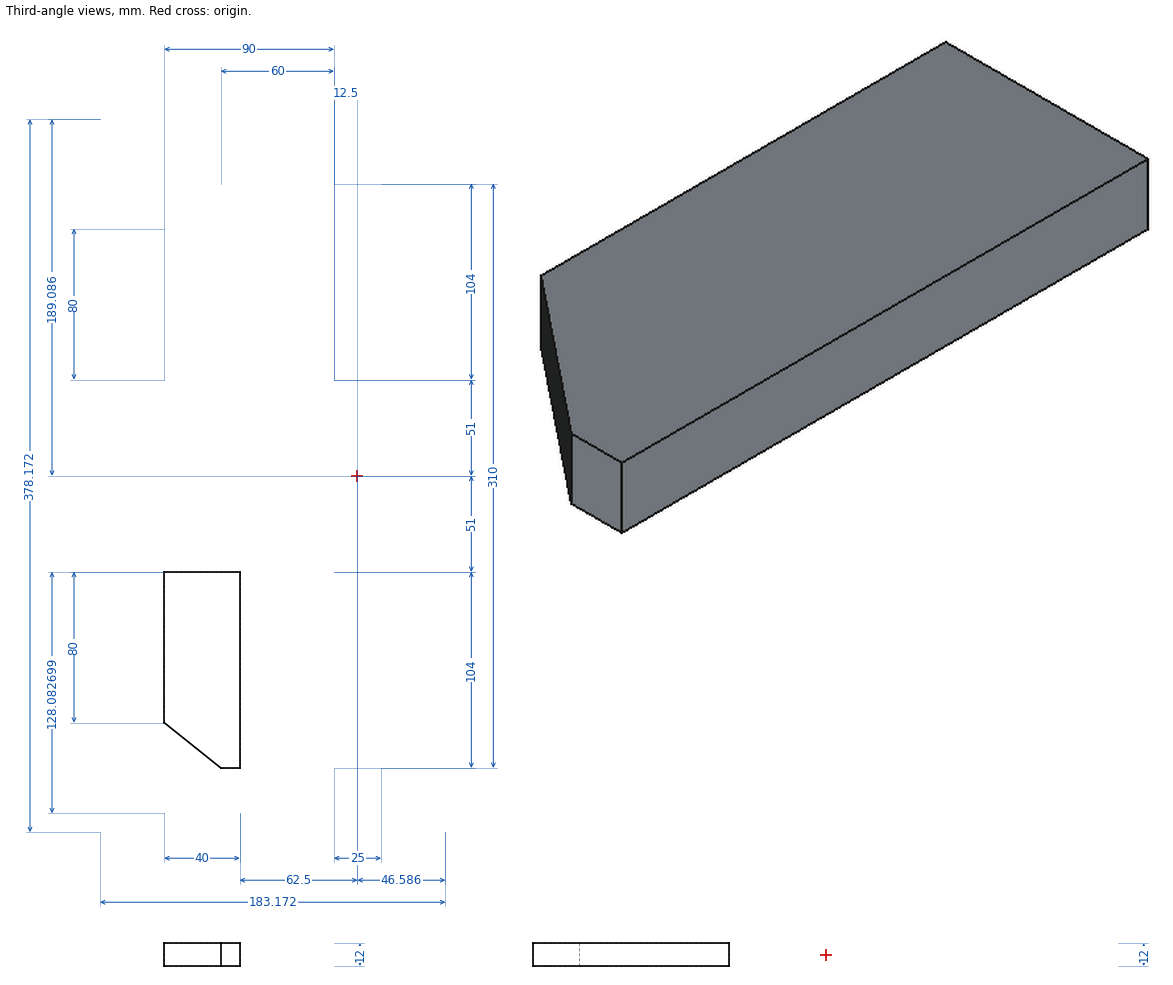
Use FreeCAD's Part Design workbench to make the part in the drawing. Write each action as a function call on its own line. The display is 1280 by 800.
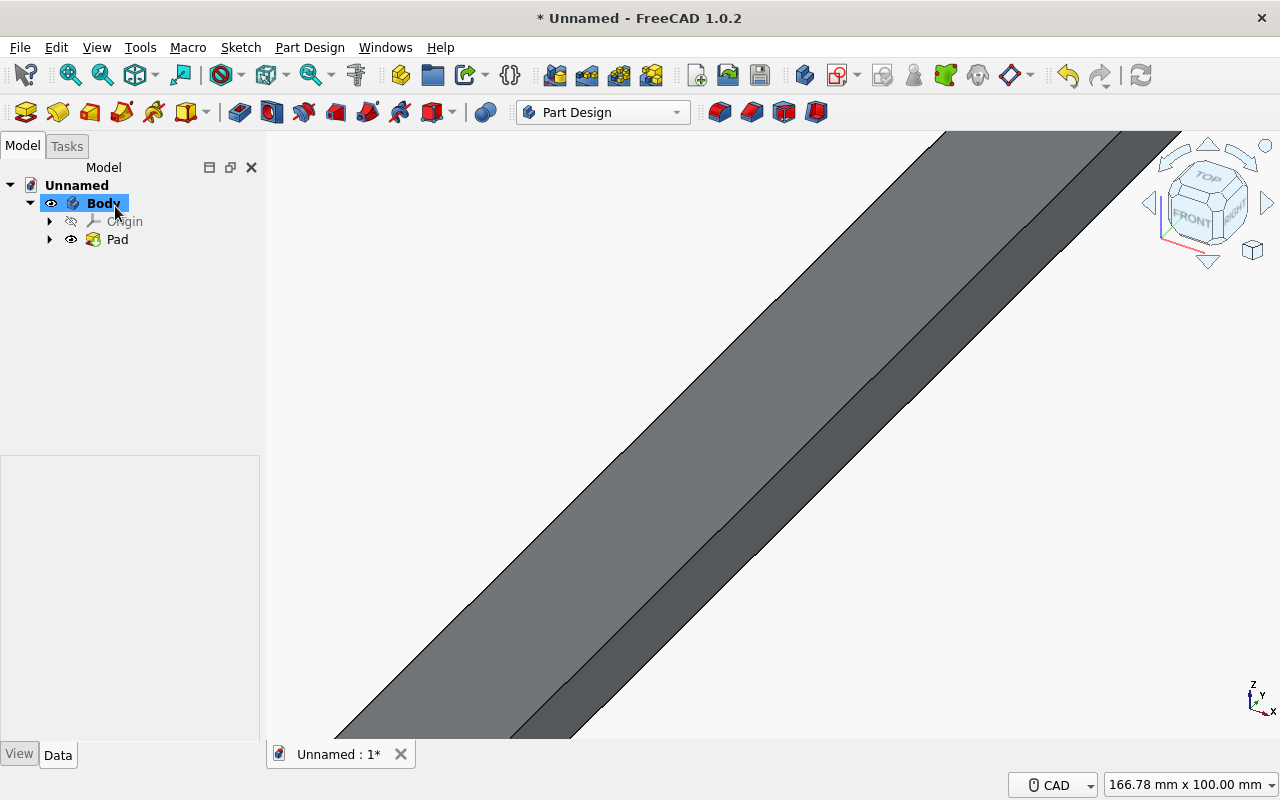
click(72, 76)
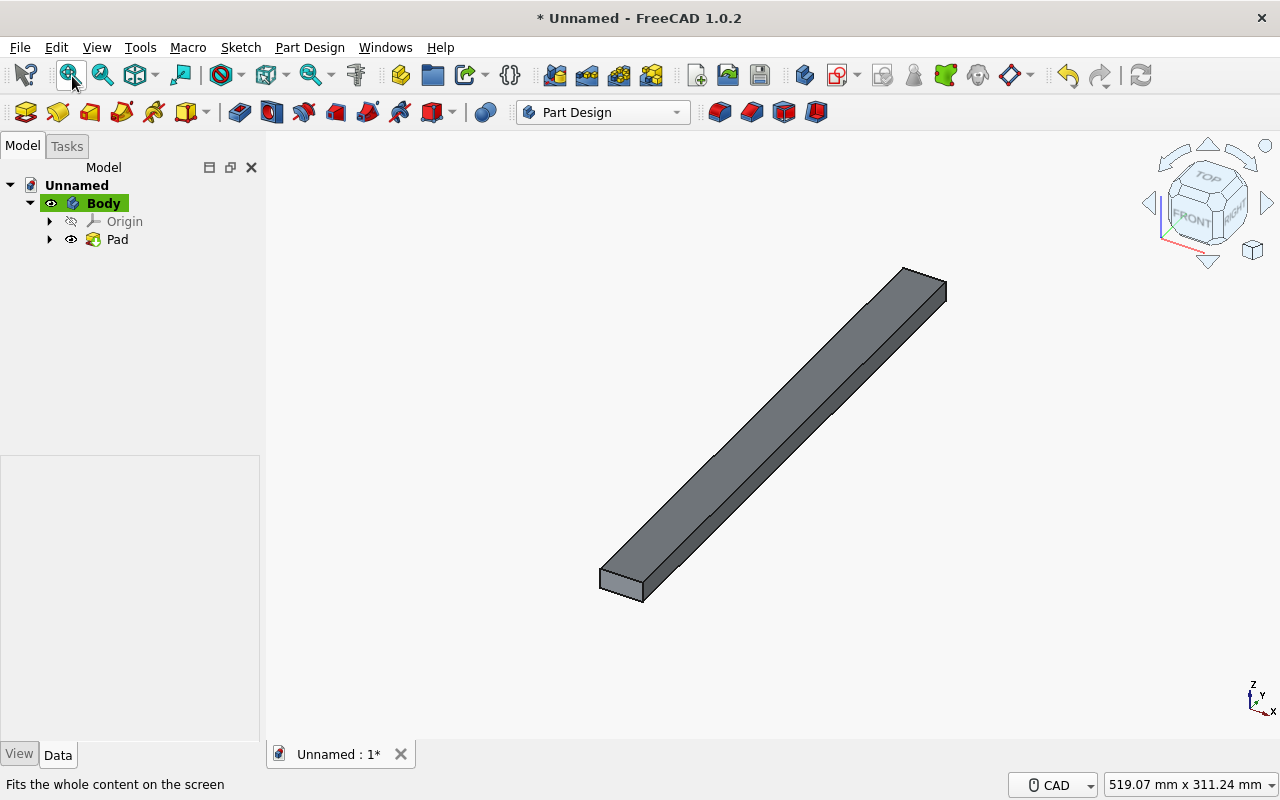
click(838, 76)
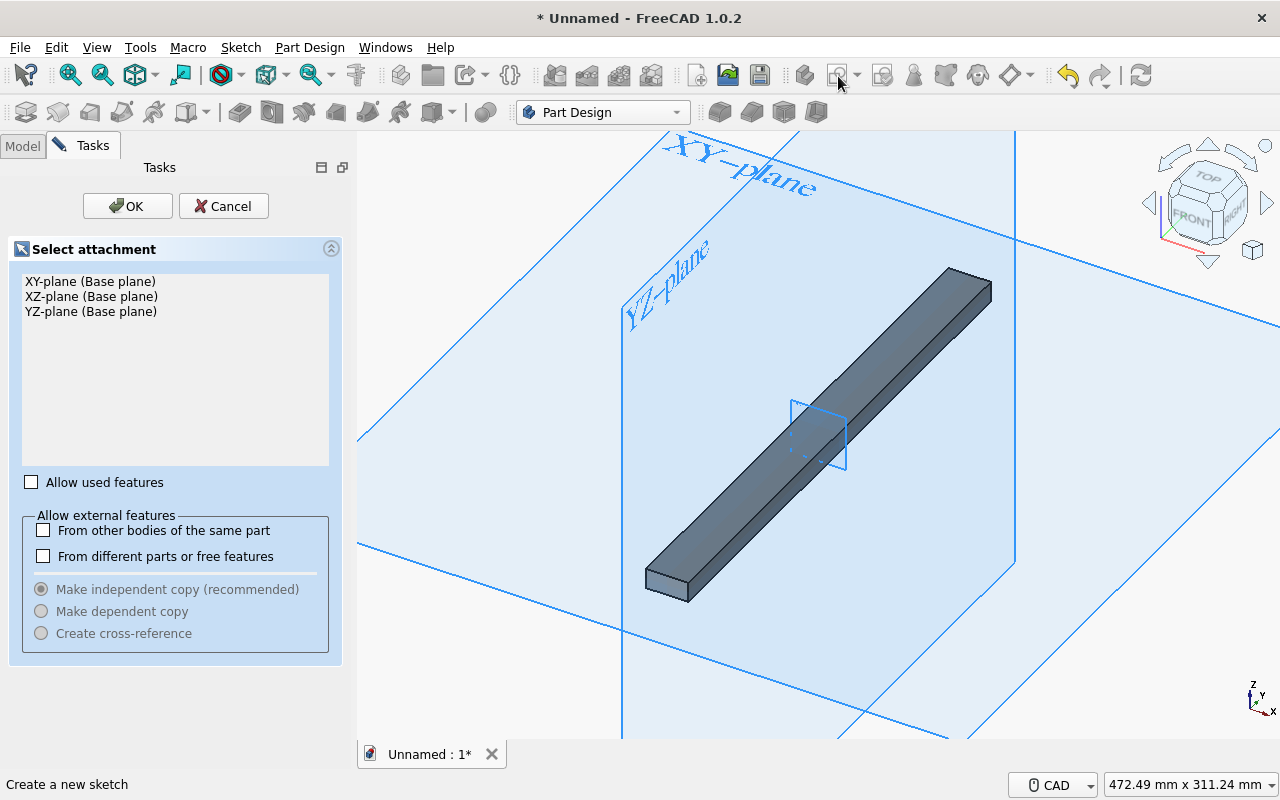
click(82, 282)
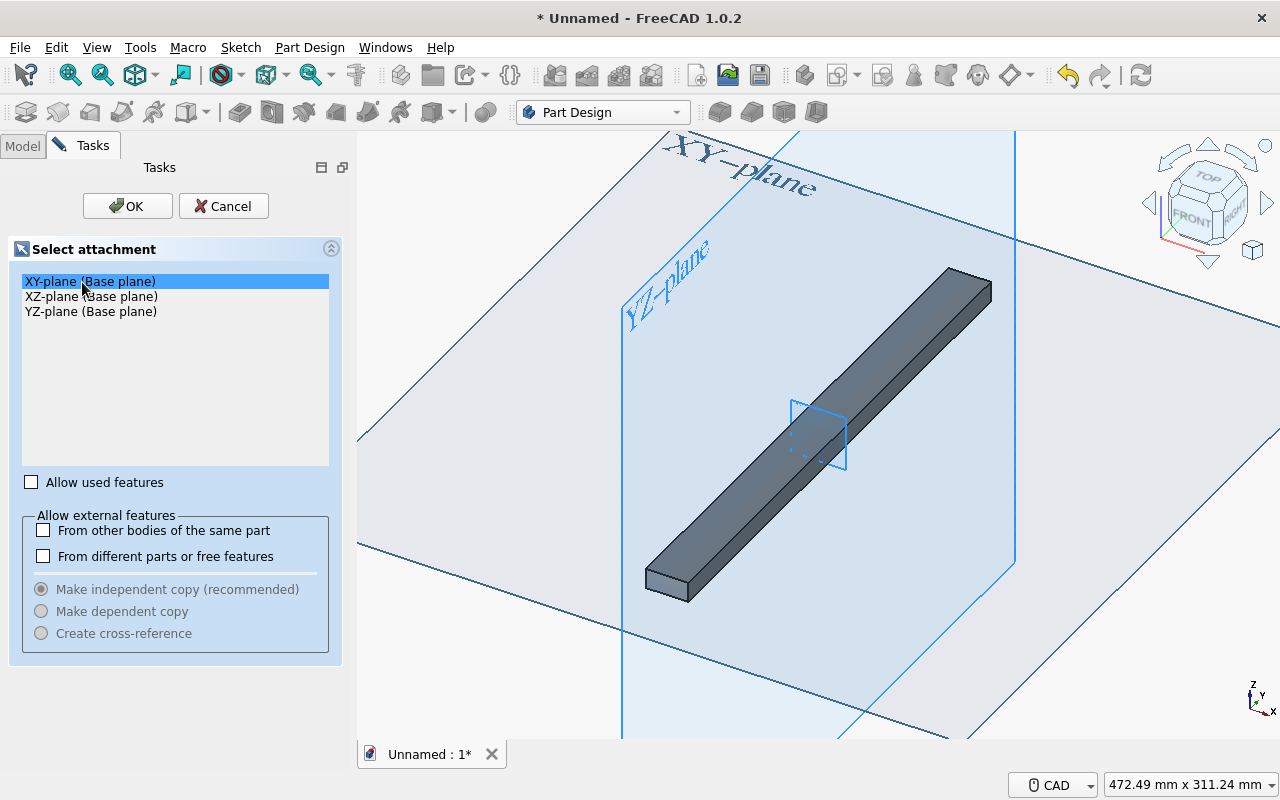
click(128, 206)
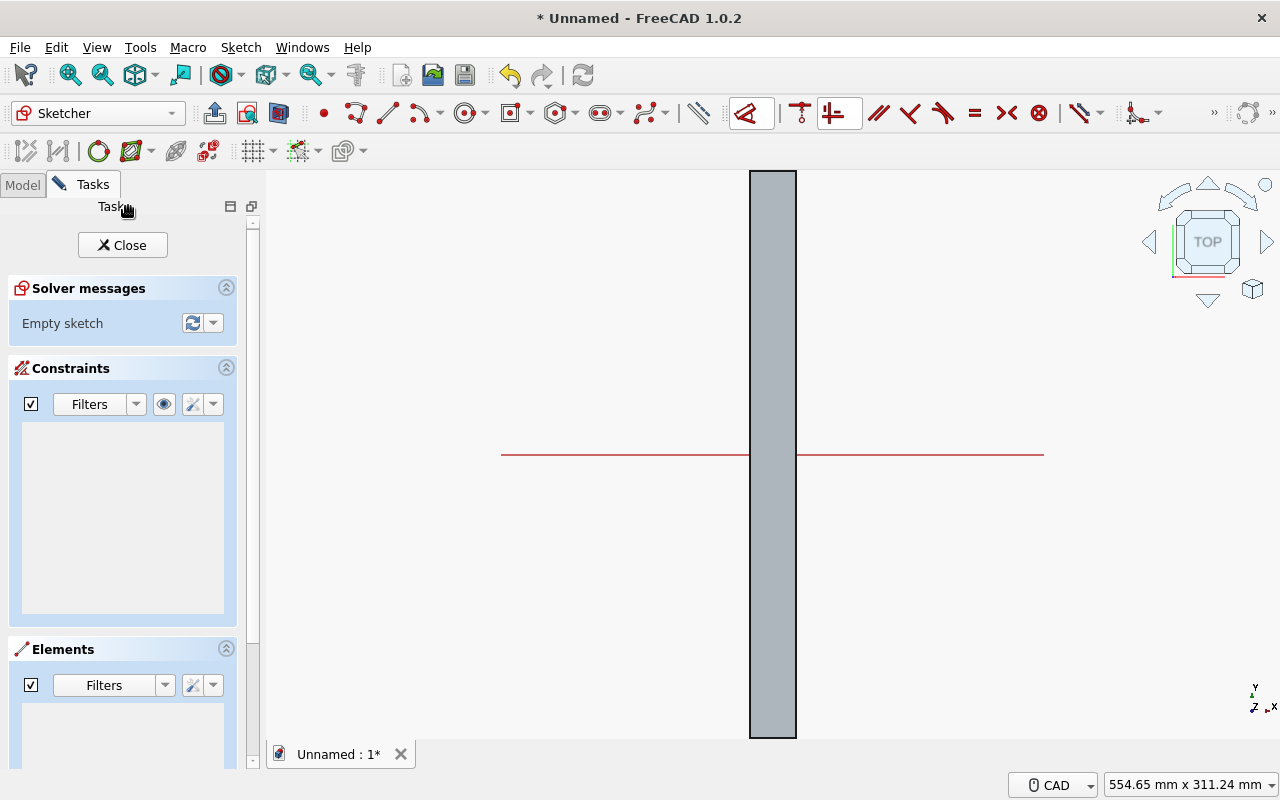
click(280, 114)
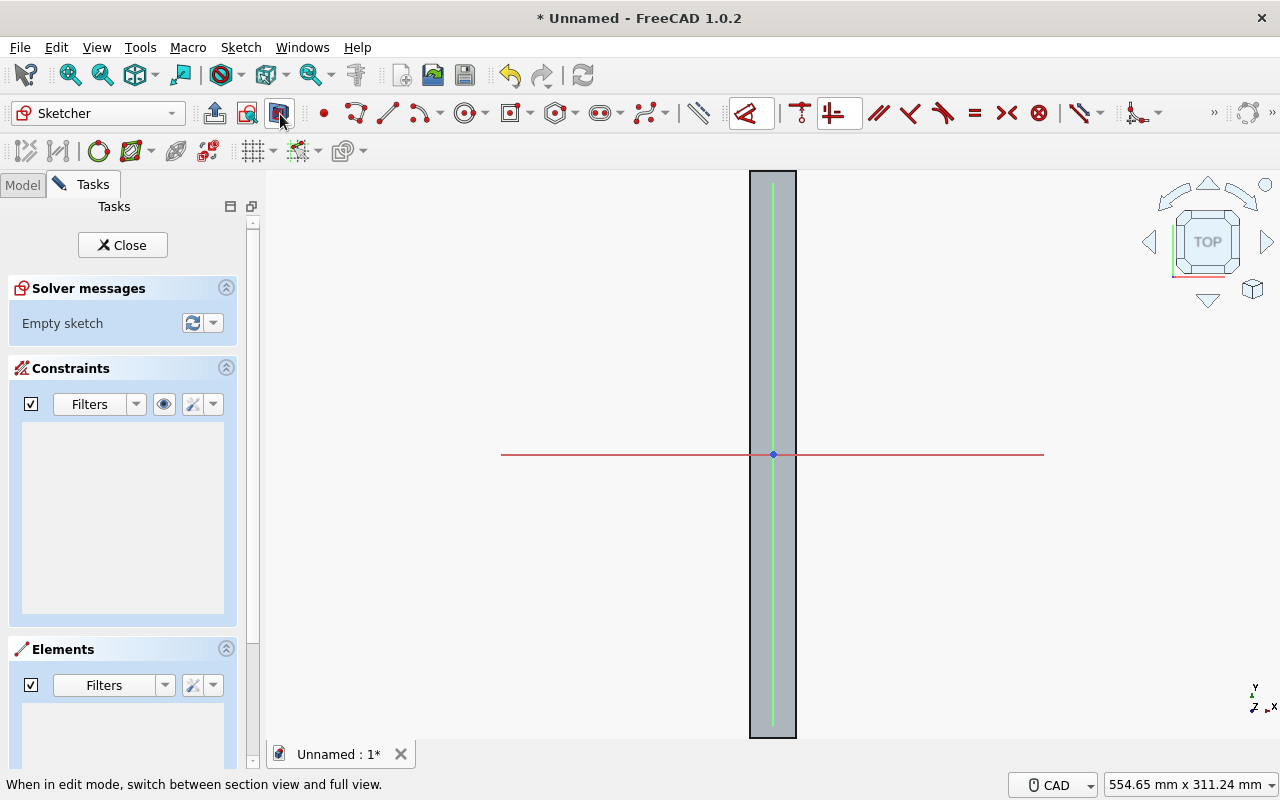
scroll(756, 455, down, 2)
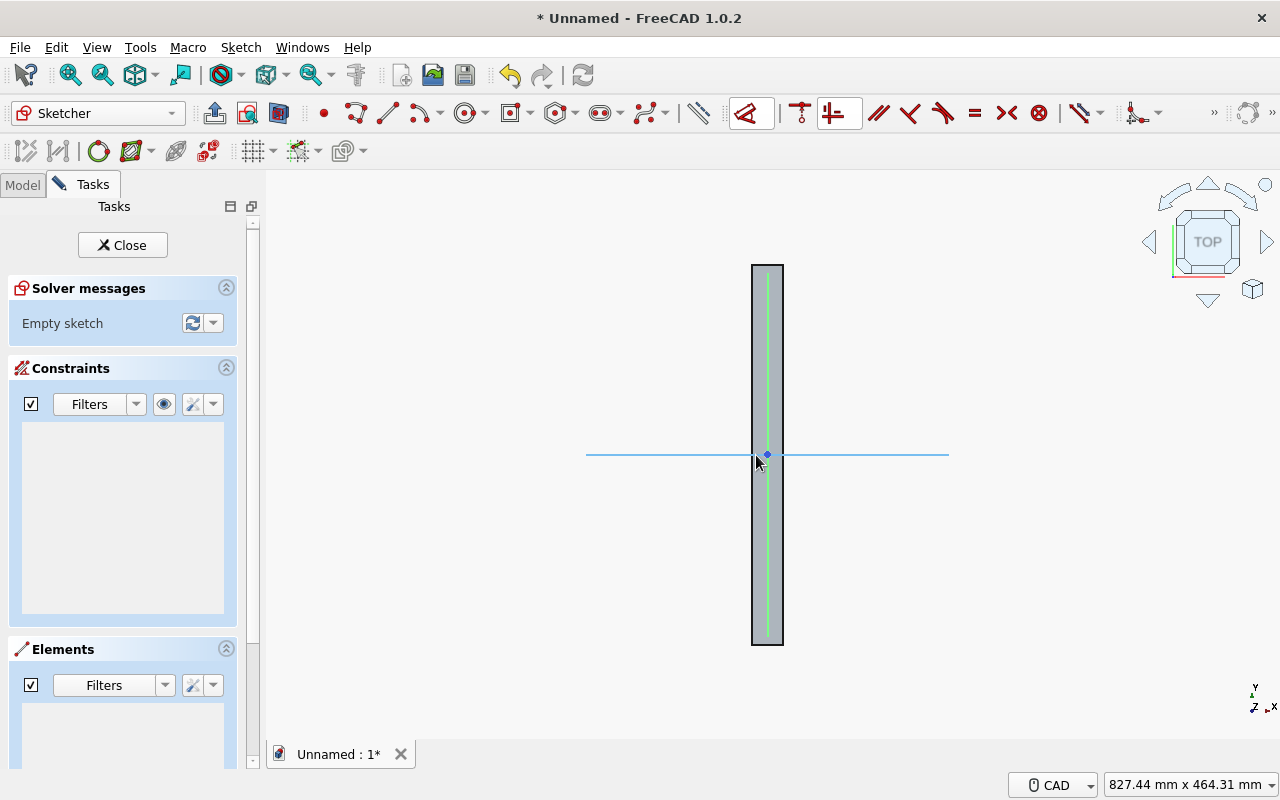
click(356, 114)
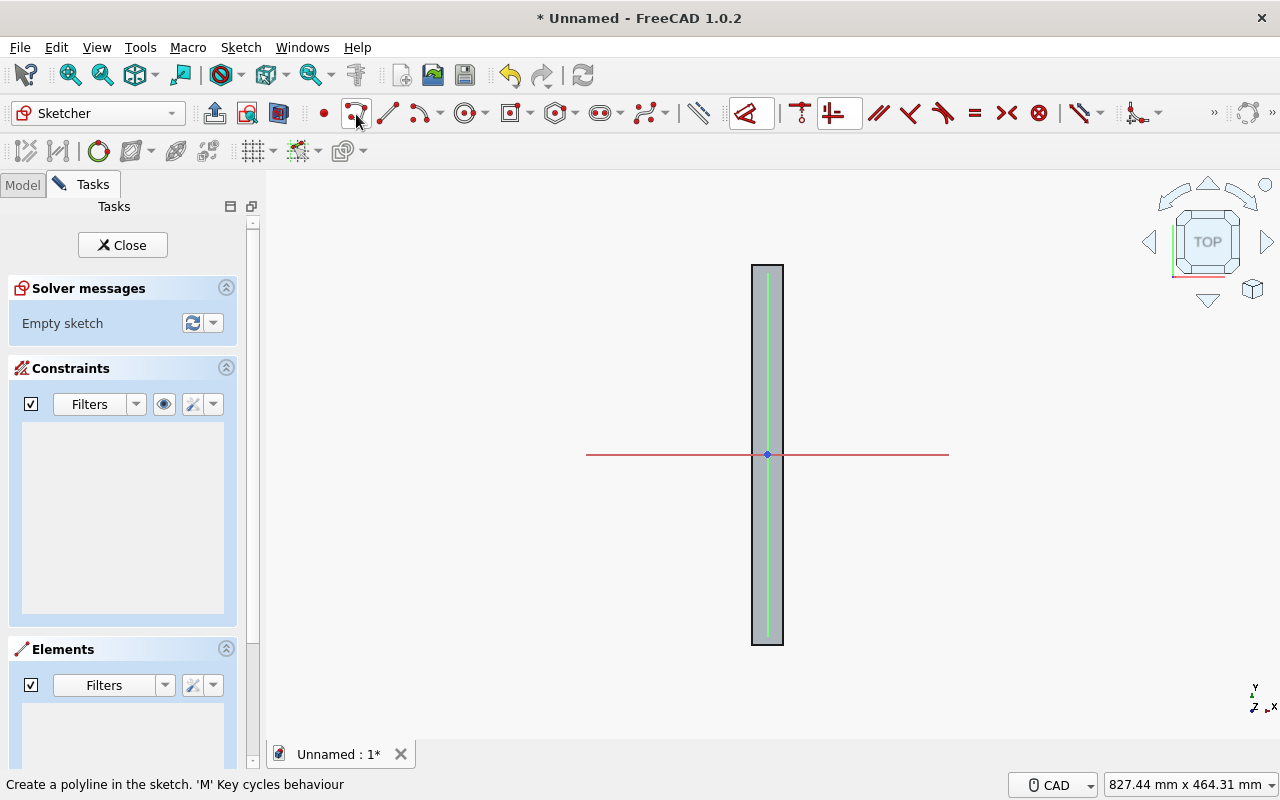
click(752, 392)
click(752, 265)
click(679, 265)
click(642, 294)
click(642, 392)
click(752, 393)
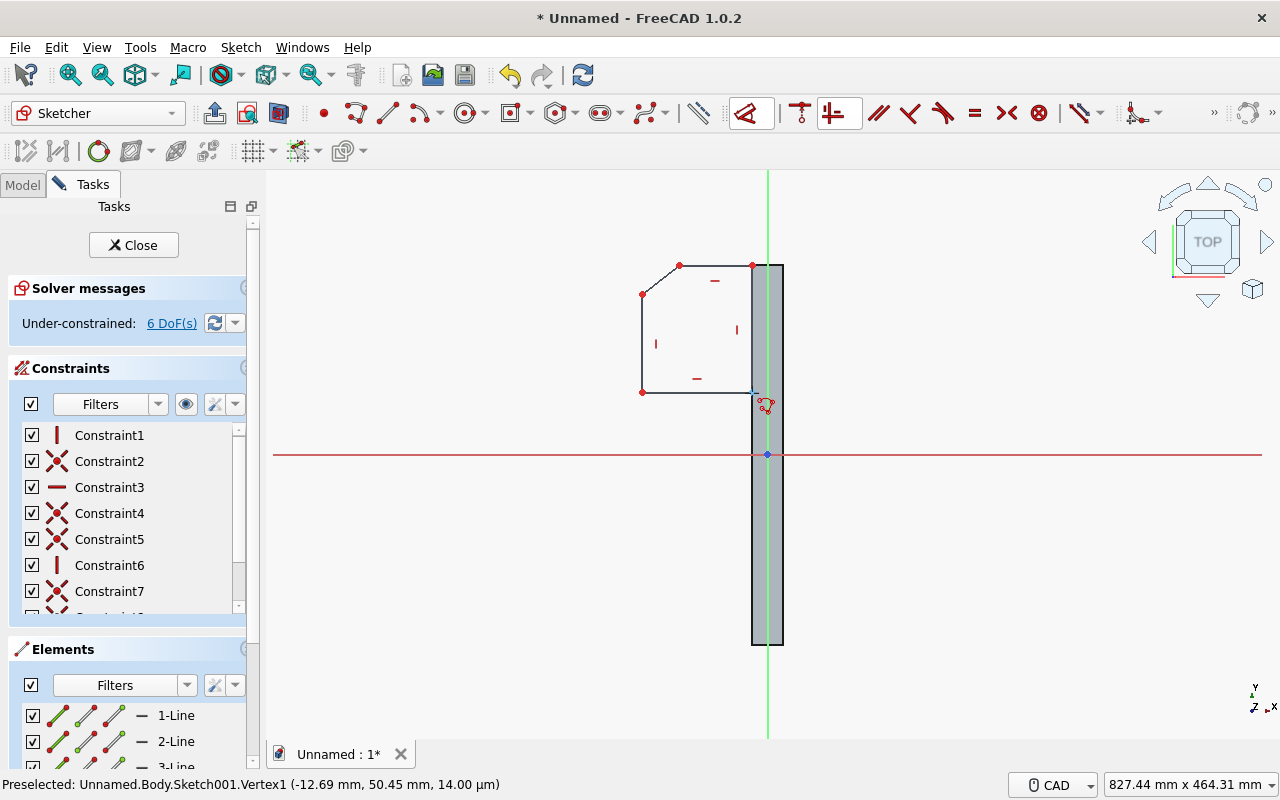
click(752, 517)
click(642, 517)
click(642, 615)
click(679, 645)
click(752, 645)
click(752, 518)
key(Escape)
key(Escape)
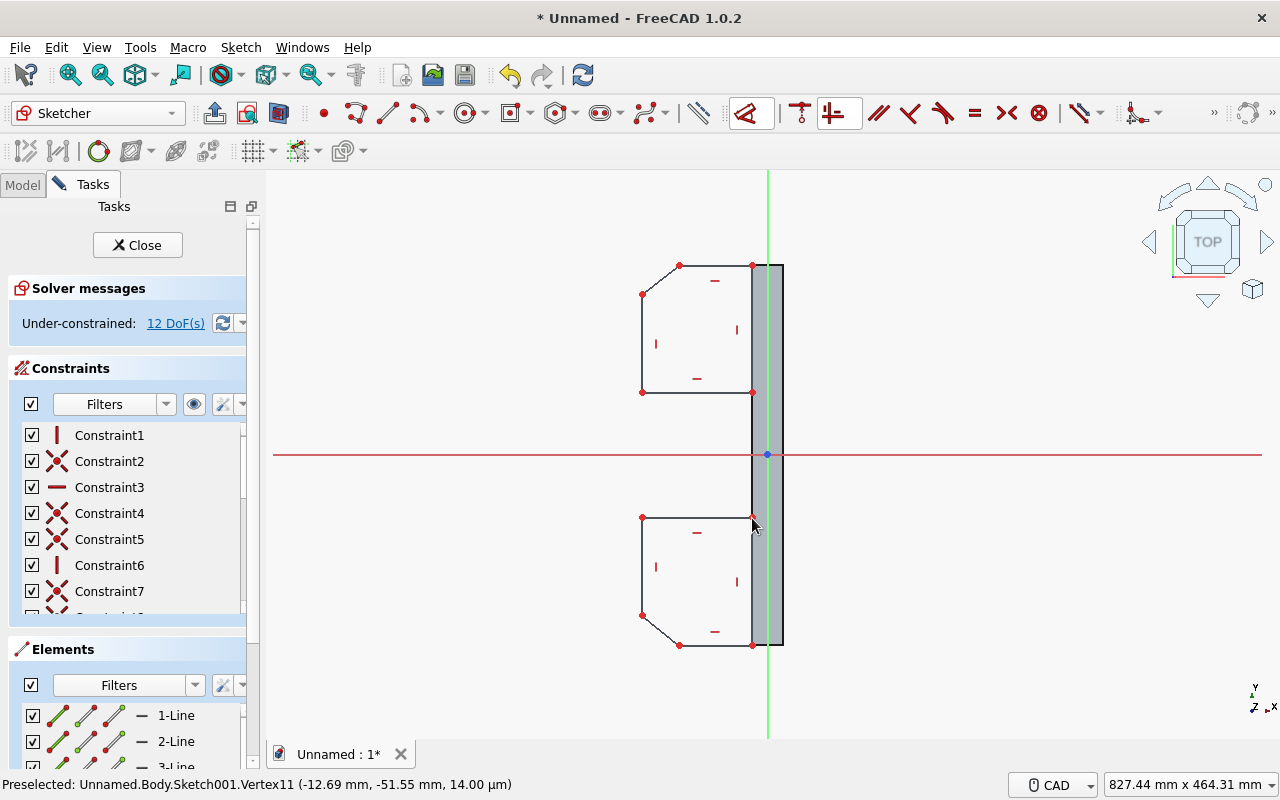
click(730, 266)